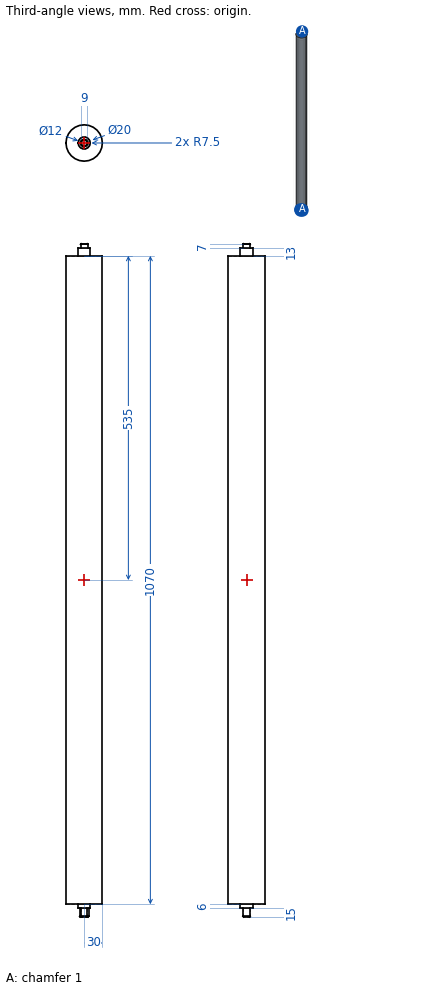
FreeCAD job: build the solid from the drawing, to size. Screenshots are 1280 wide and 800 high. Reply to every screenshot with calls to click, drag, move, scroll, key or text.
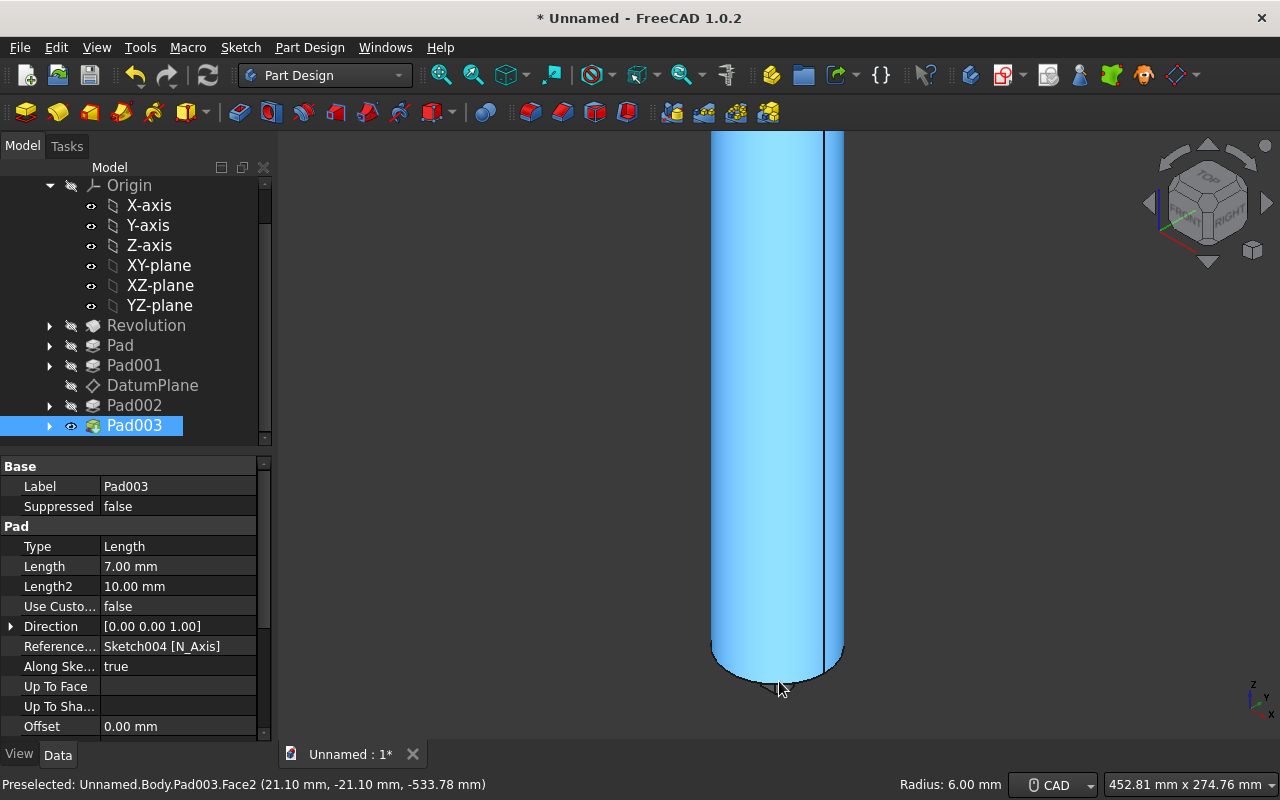
key(v)
key(f)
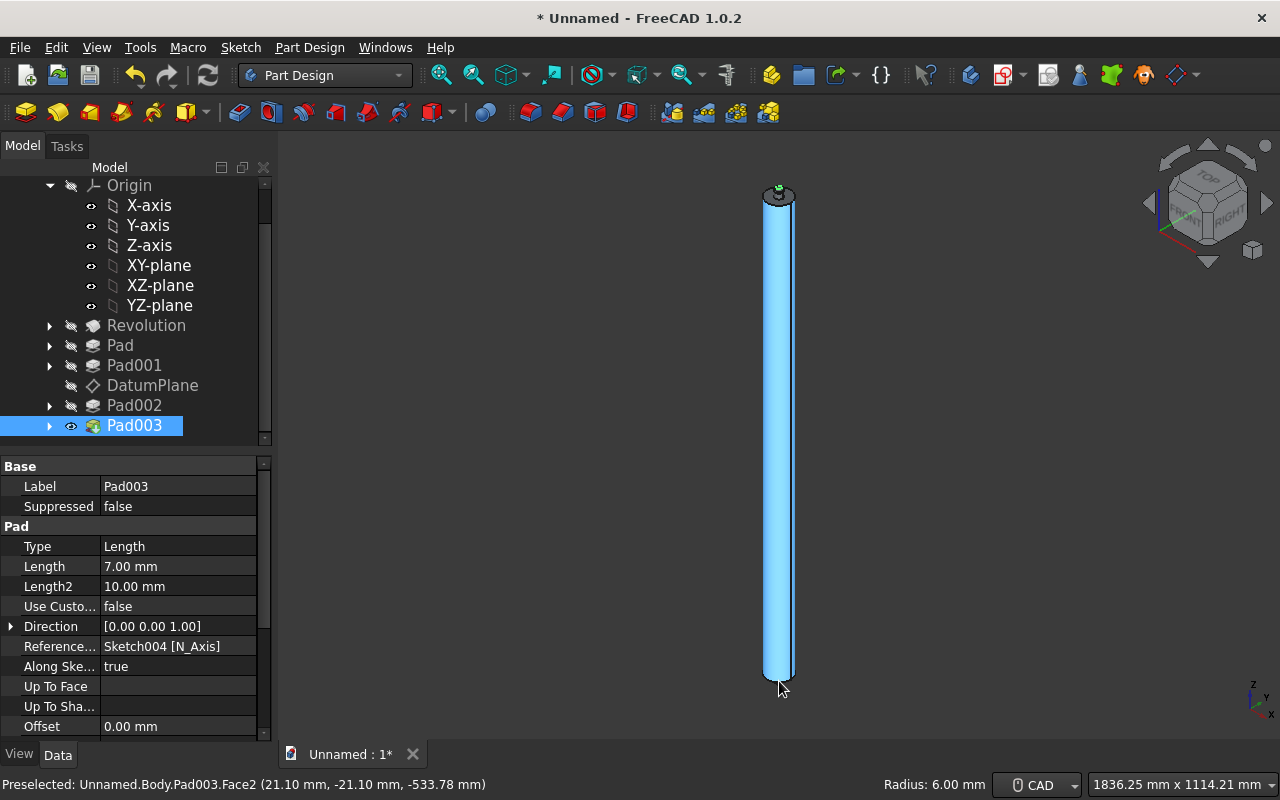
key(2)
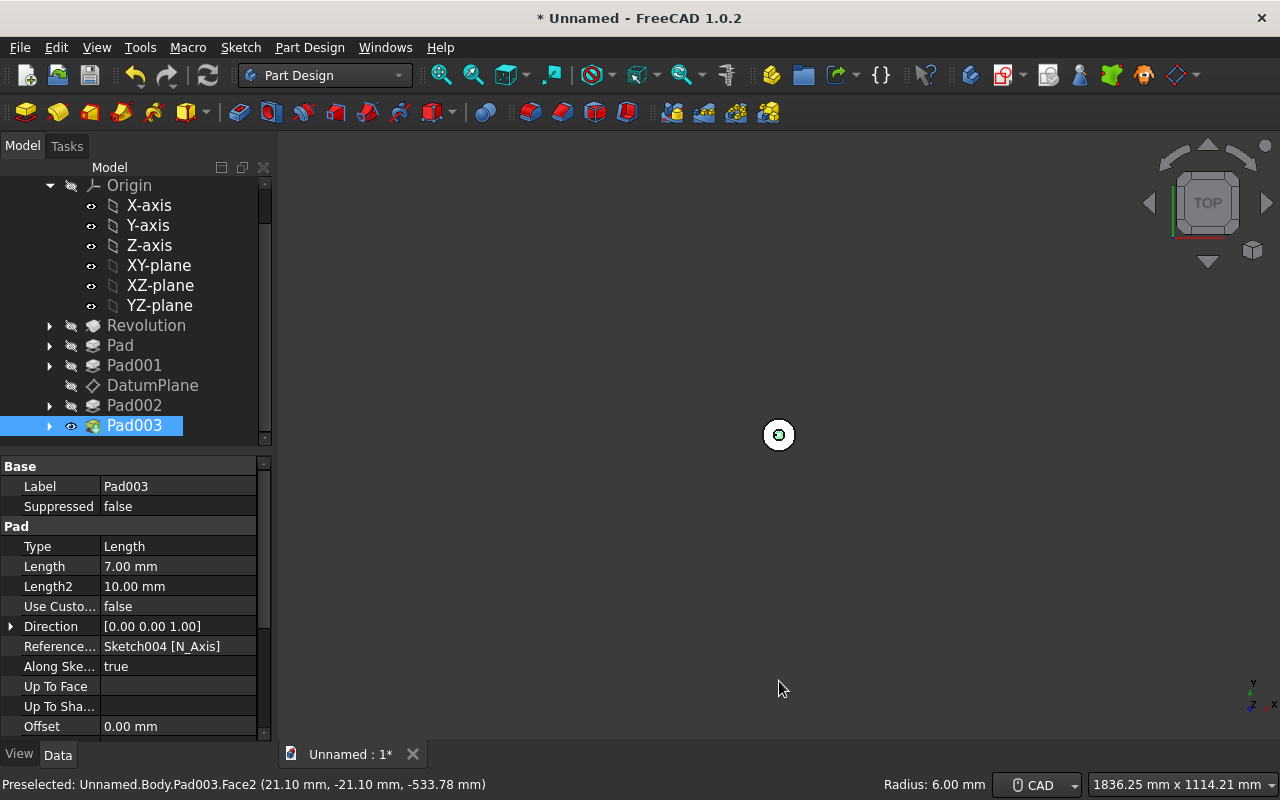
click(442, 76)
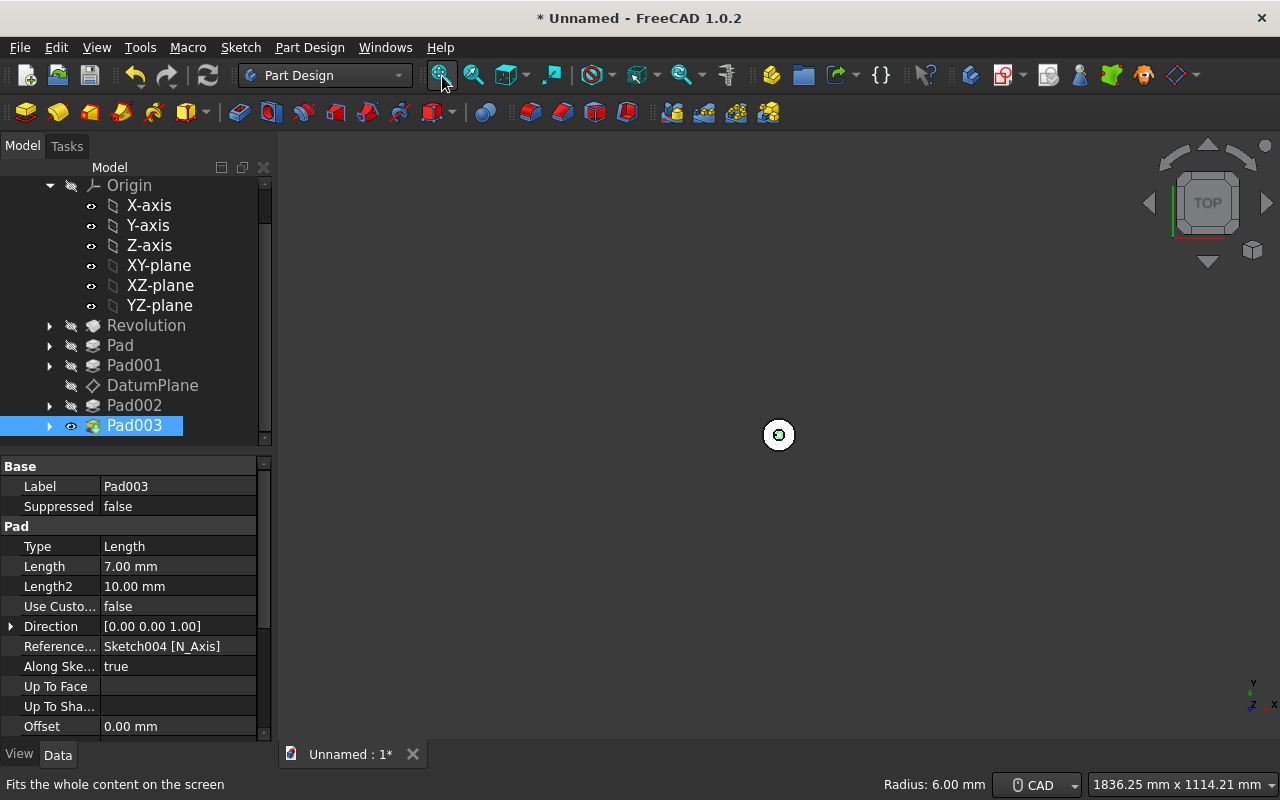
scroll(779, 434, up, 7)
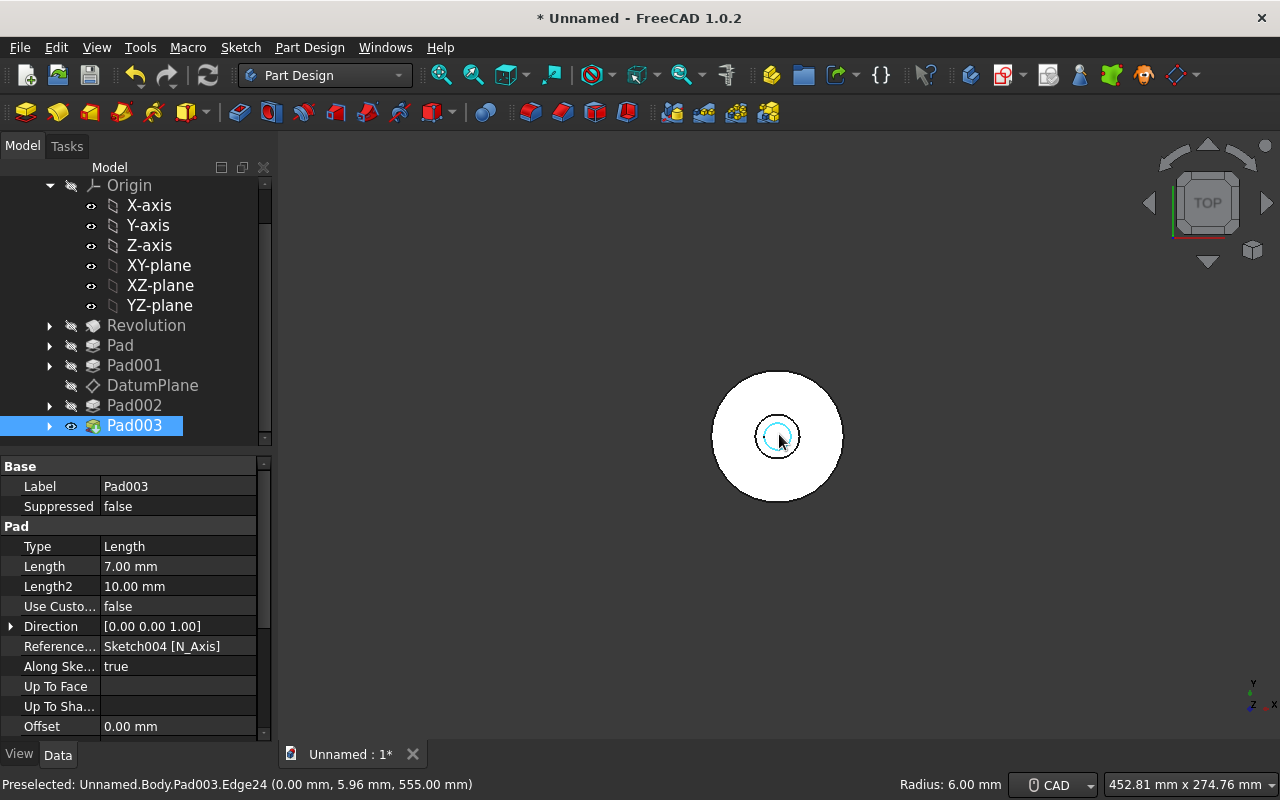
key(v)
key(f)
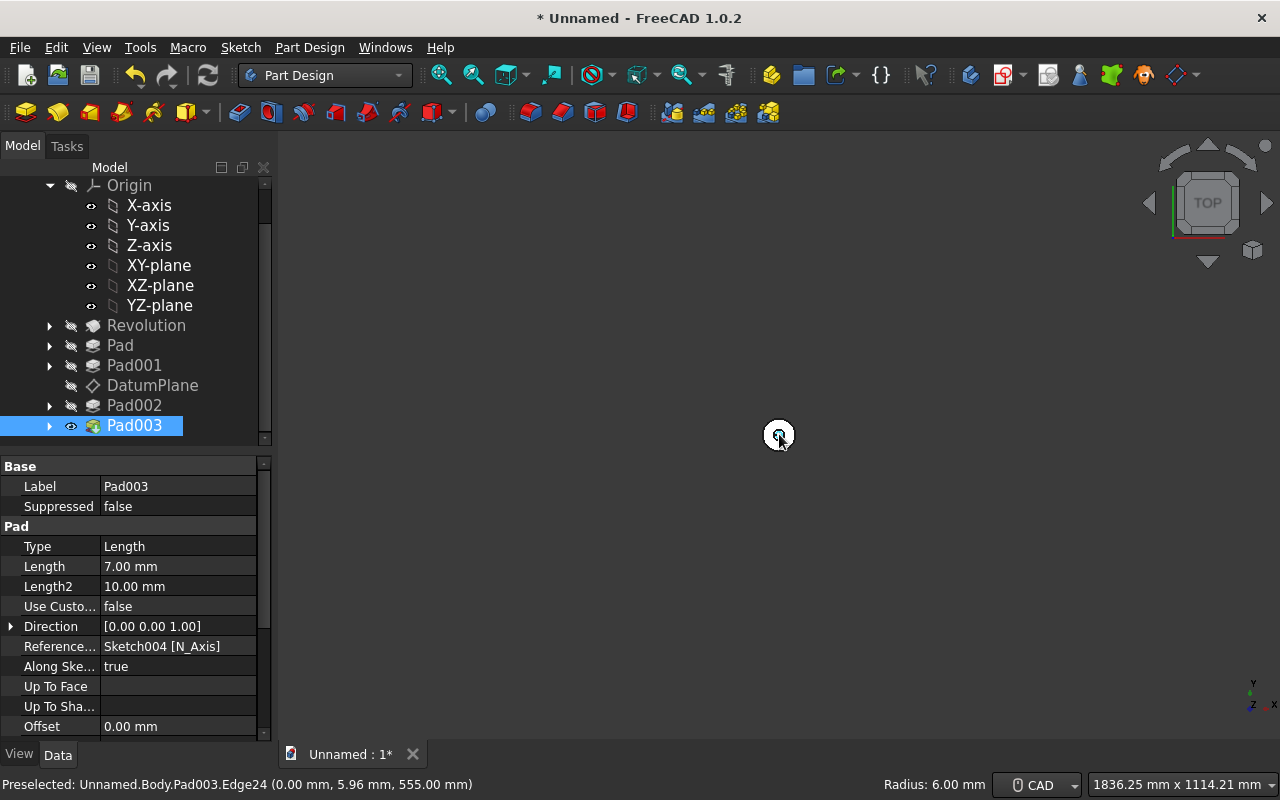
key(1)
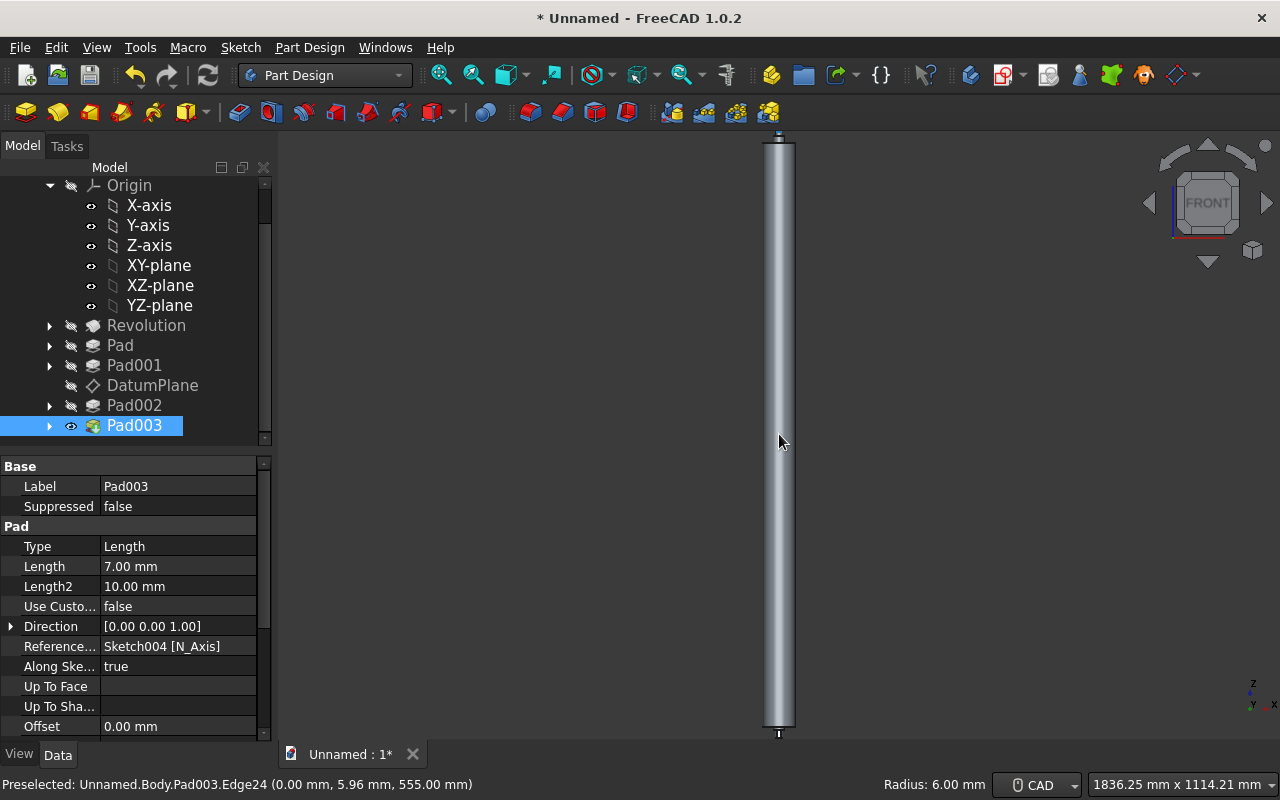
key(3)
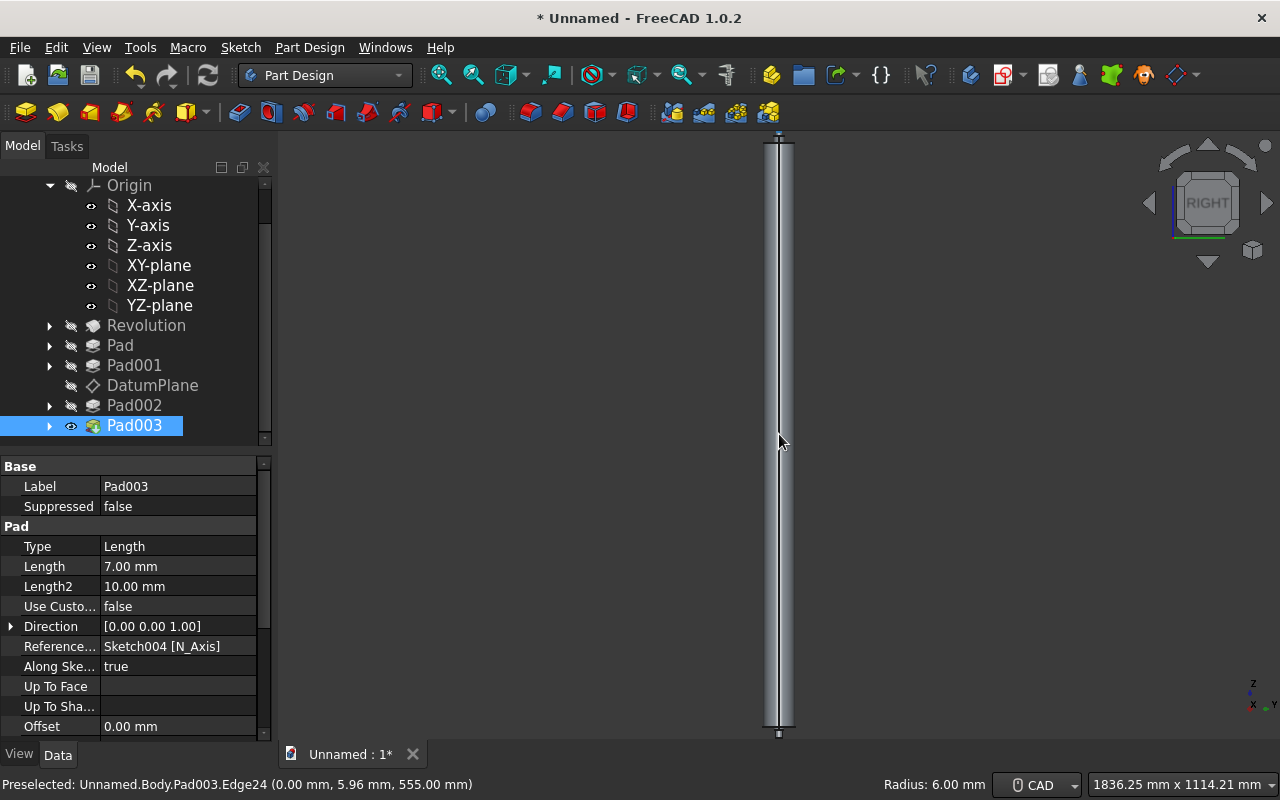
key(5)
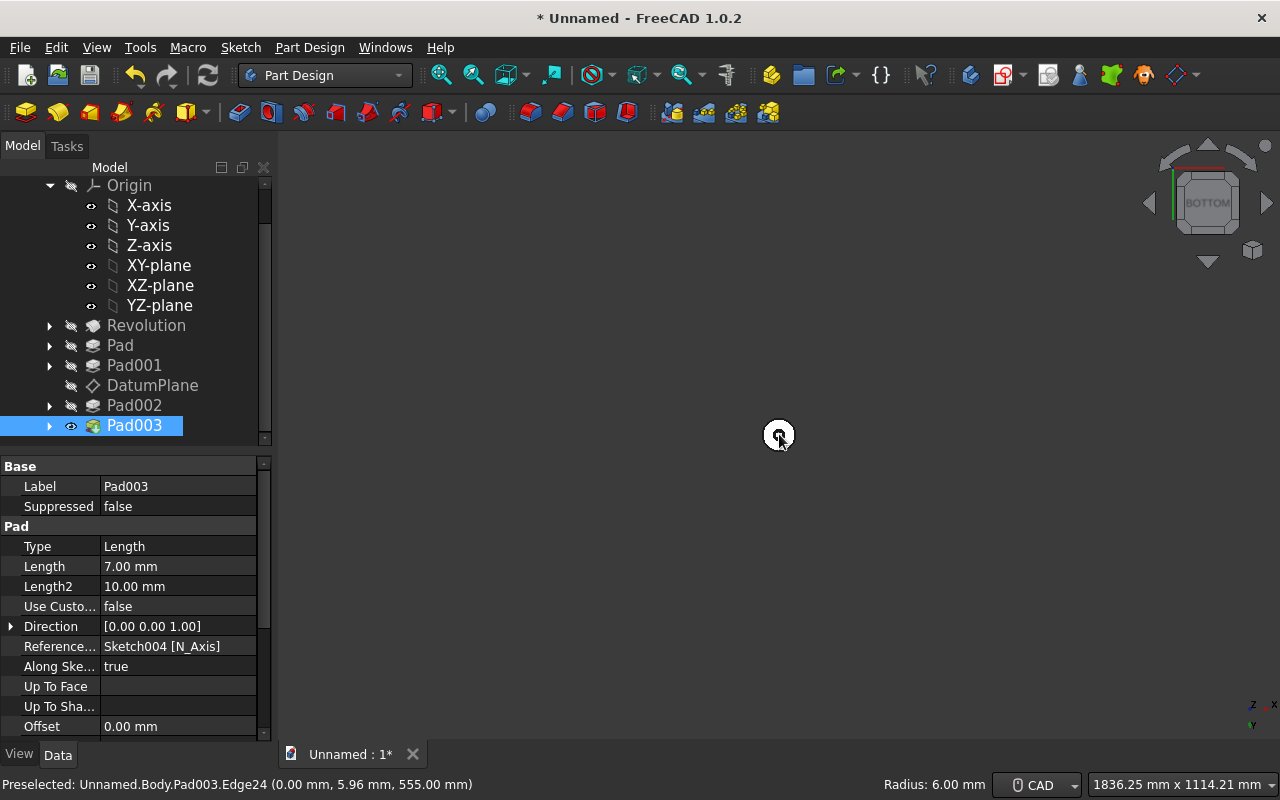
key(v)
key(f)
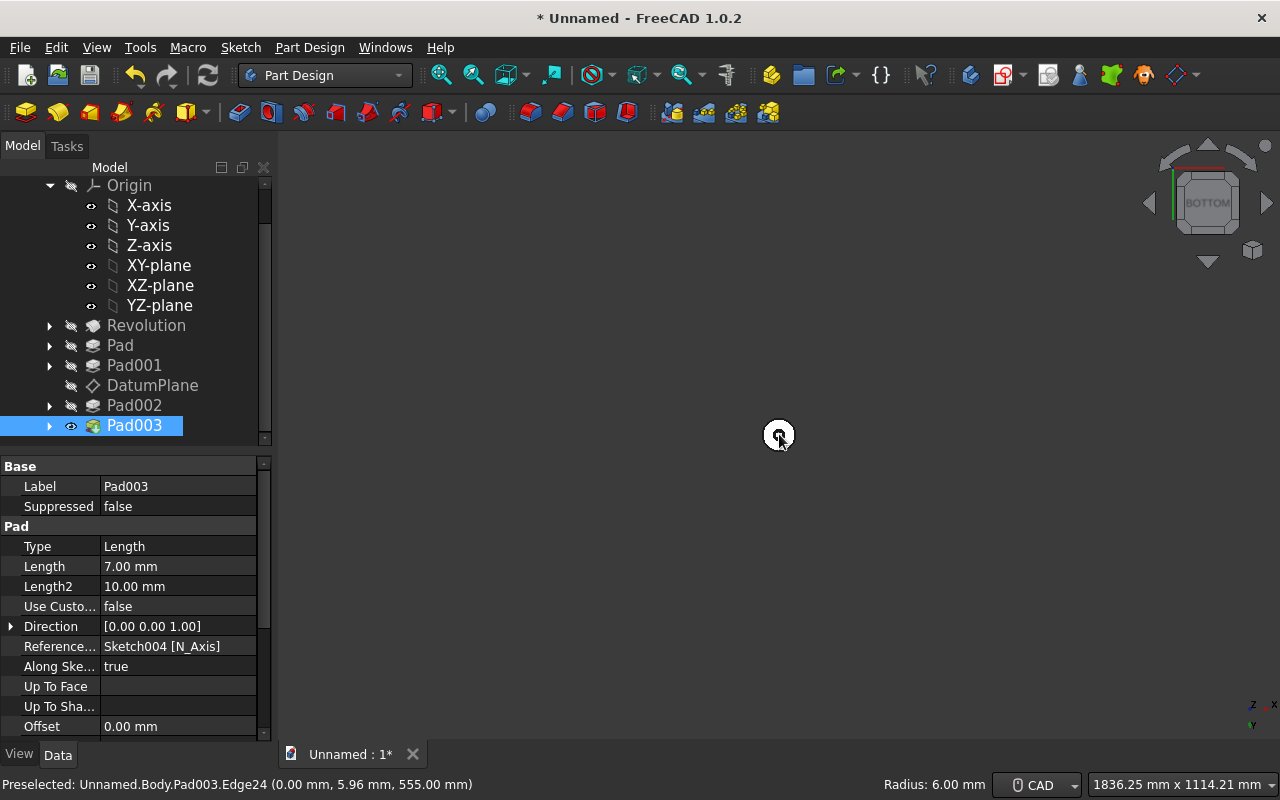
scroll(779, 434, up, 7)